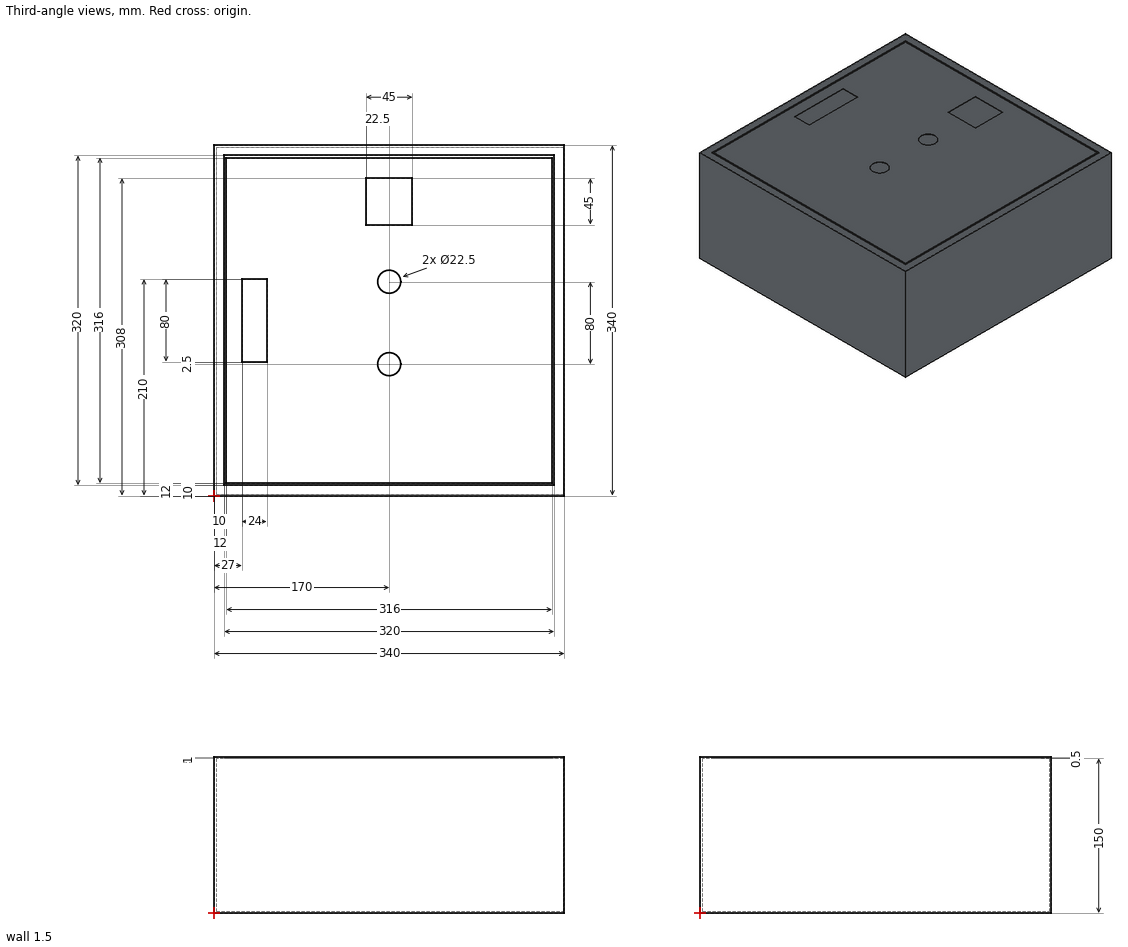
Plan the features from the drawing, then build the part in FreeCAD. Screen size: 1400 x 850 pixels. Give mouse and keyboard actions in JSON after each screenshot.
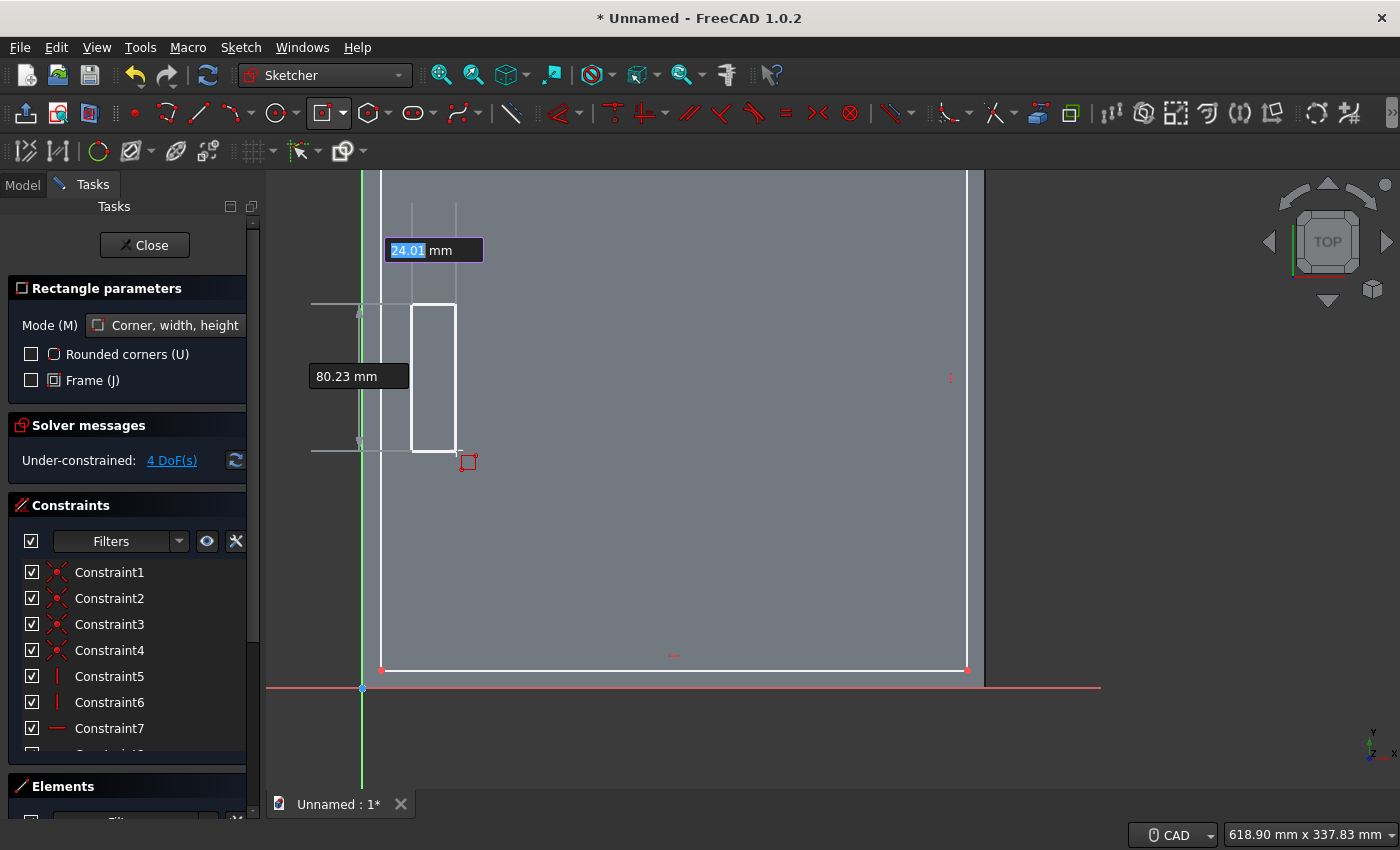
{"action": "type", "text": "24"}
{"action": "key", "text": "Tab"}
{"action": "type", "text": "80"}
{"action": "key", "text": "Return"}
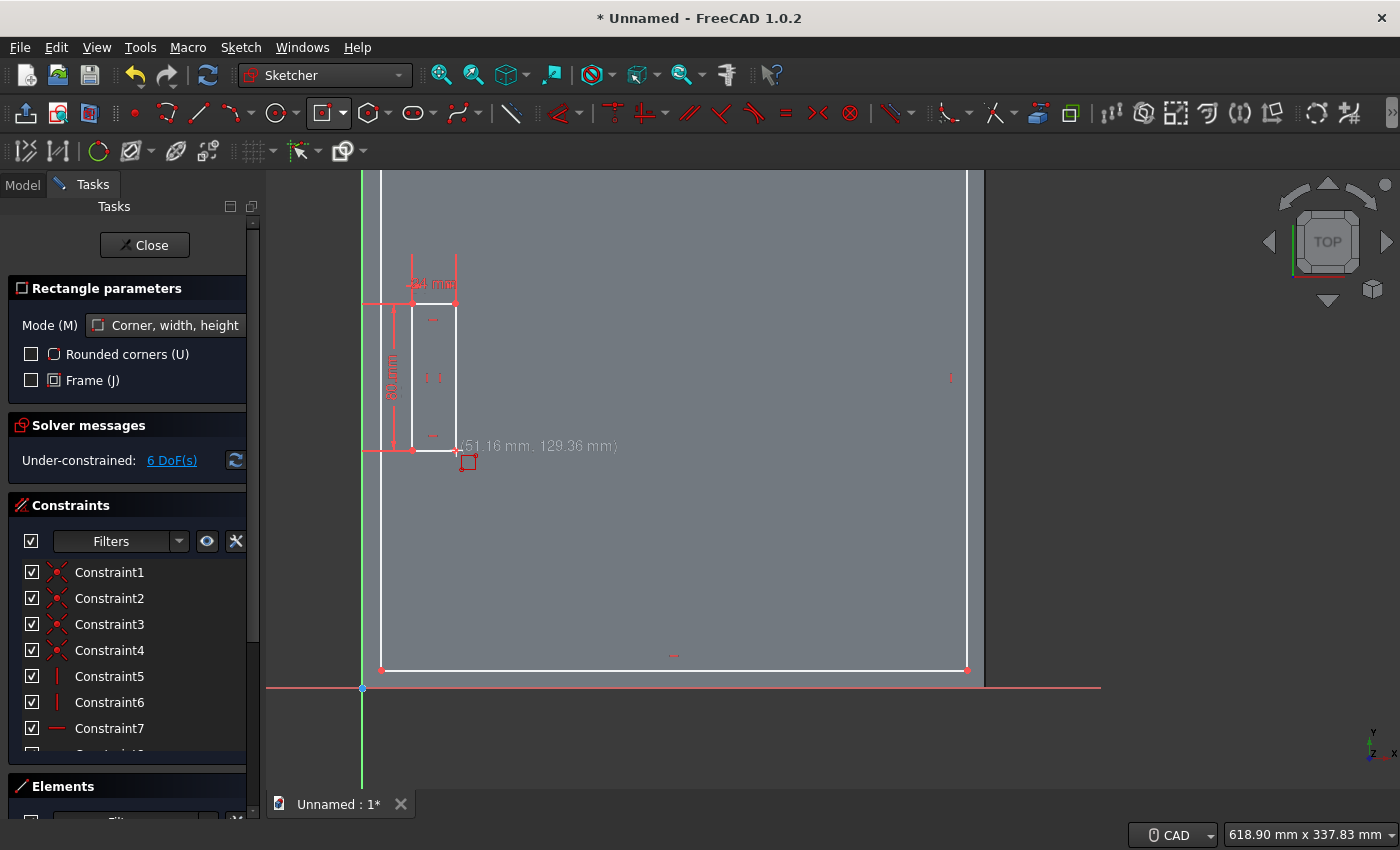
{"action": "scroll", "coordinate": [968, 670], "scroll_direction": "down", "scroll_amount": 2}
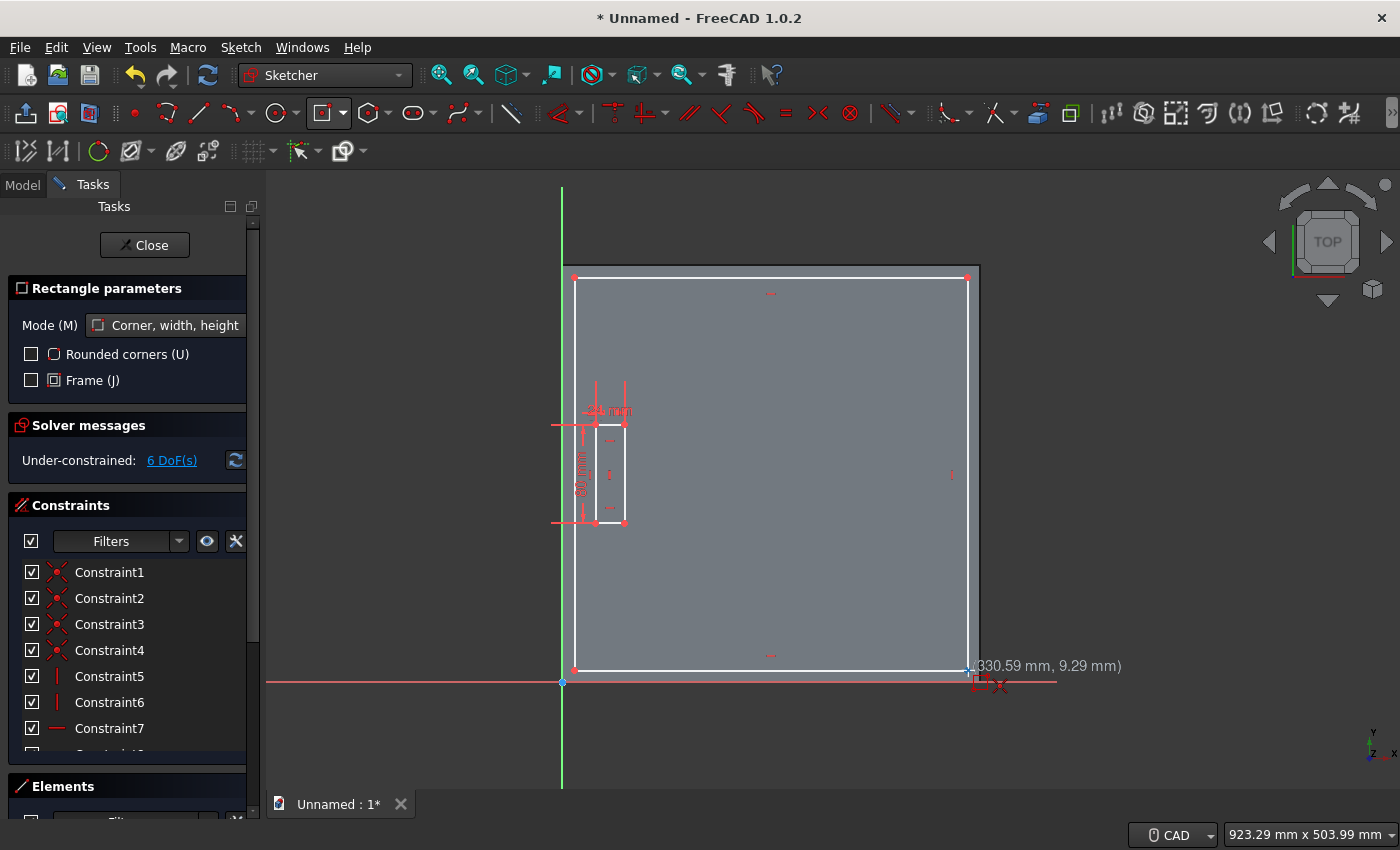
{"action": "left_click", "coordinate": [743, 304]}
{"action": "mouse_move", "coordinate": [799, 359]}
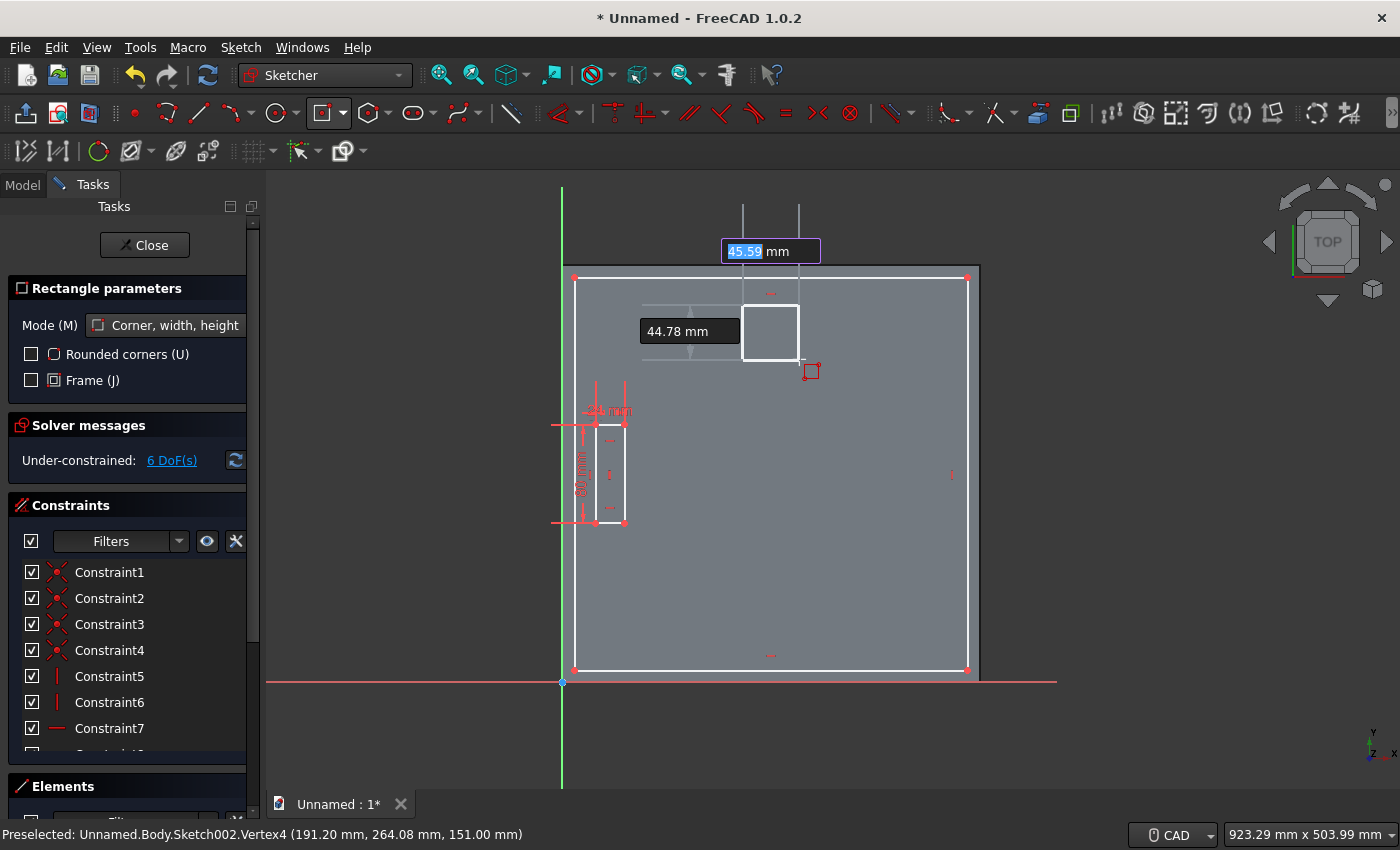
{"action": "type", "text": "45"}
{"action": "key", "text": "Tab"}
{"action": "type", "text": "45"}
{"action": "key", "text": "Return"}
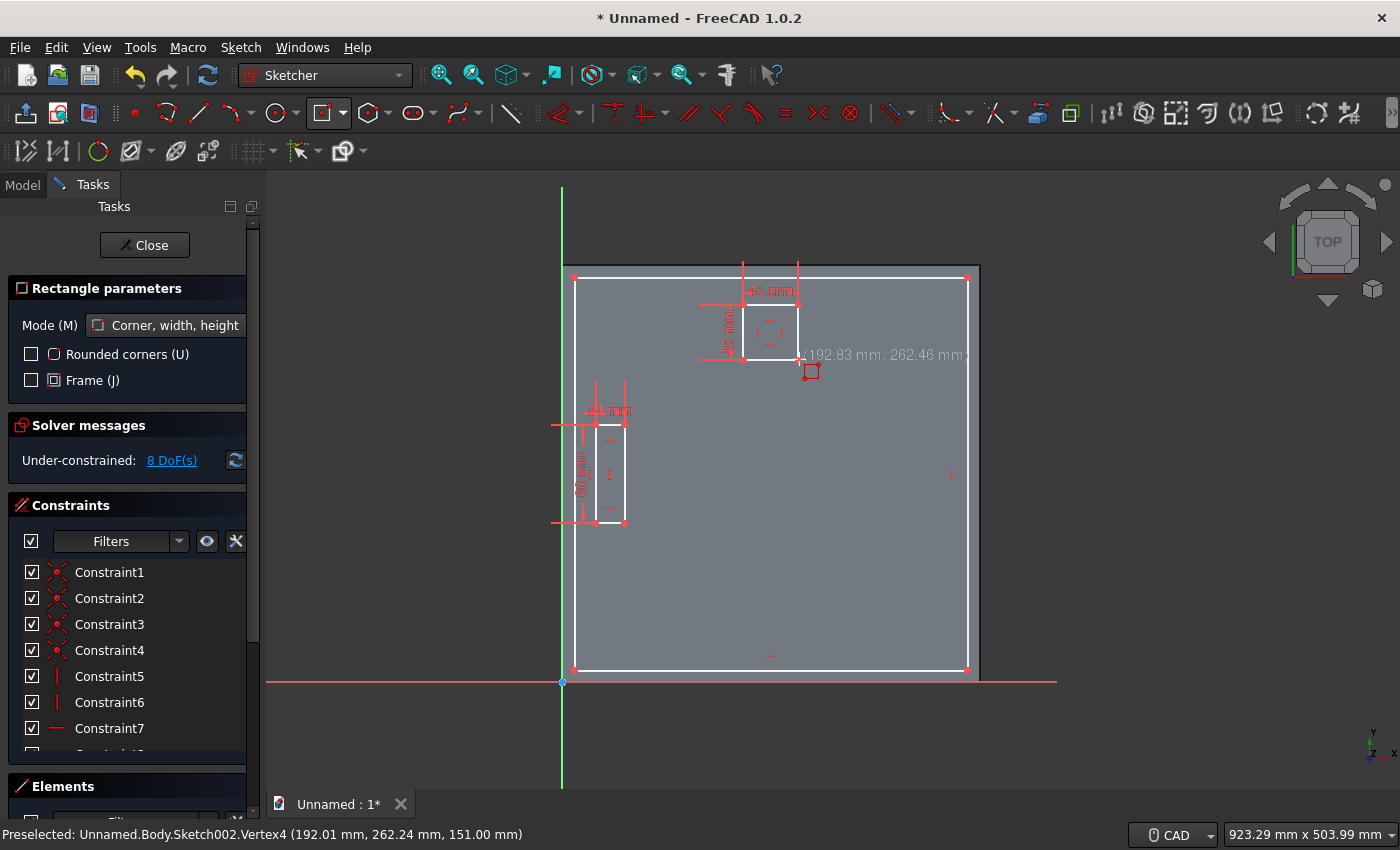
{"action": "scroll", "coordinate": [577, 279], "scroll_direction": "up", "scroll_amount": 10}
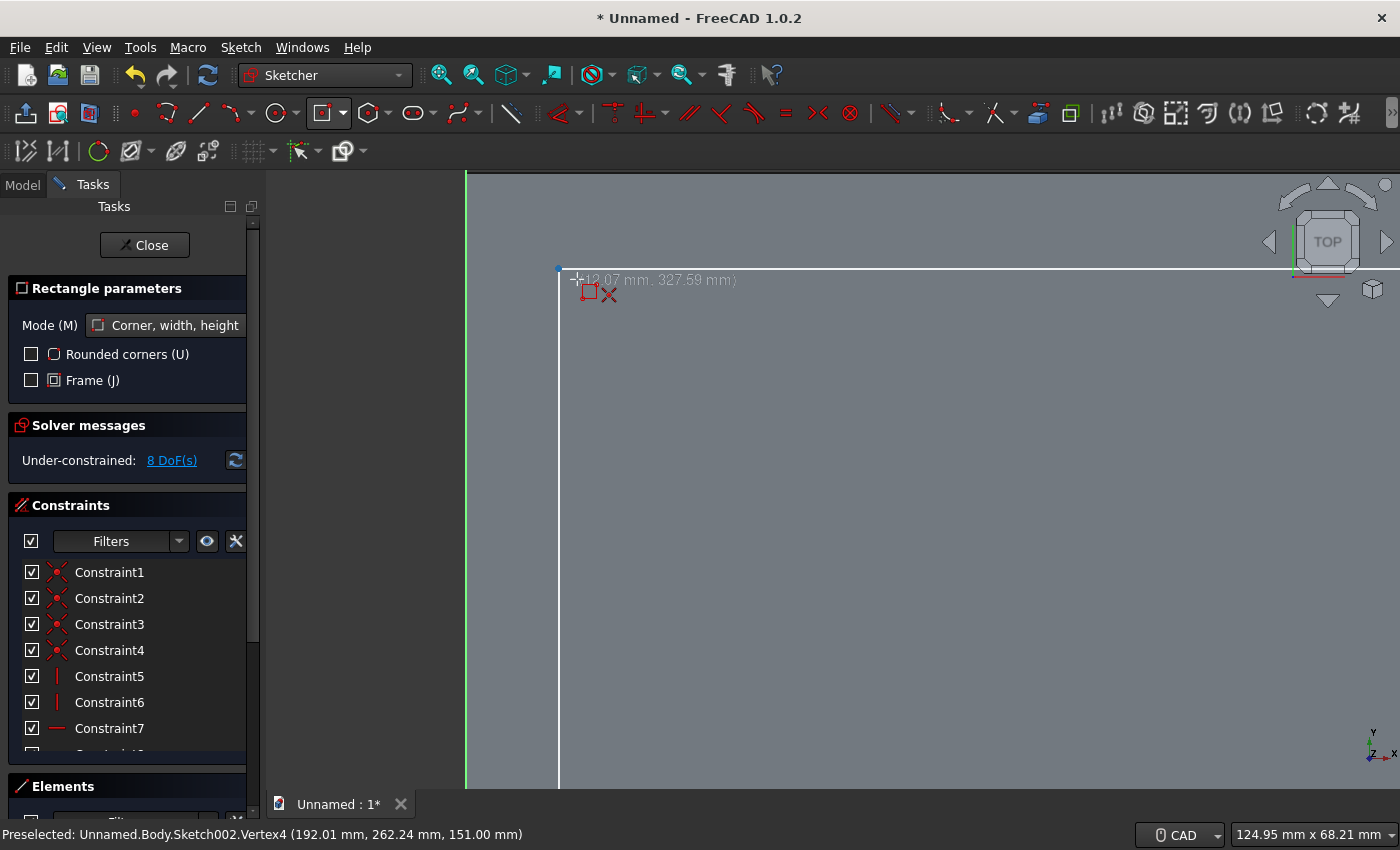
{"action": "left_click", "coordinate": [575, 282]}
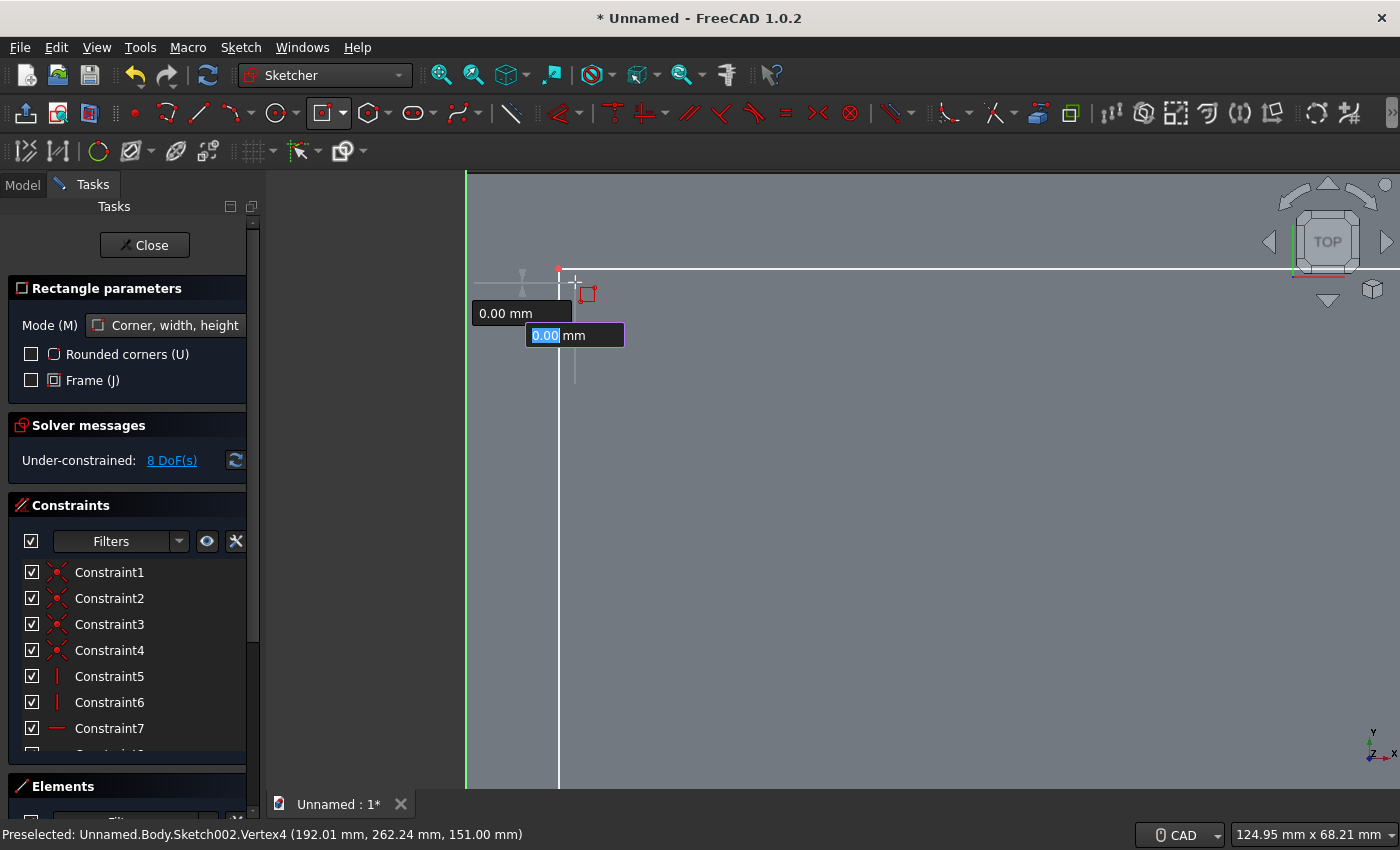
{"action": "scroll", "coordinate": [577, 279], "scroll_direction": "down", "scroll_amount": 10}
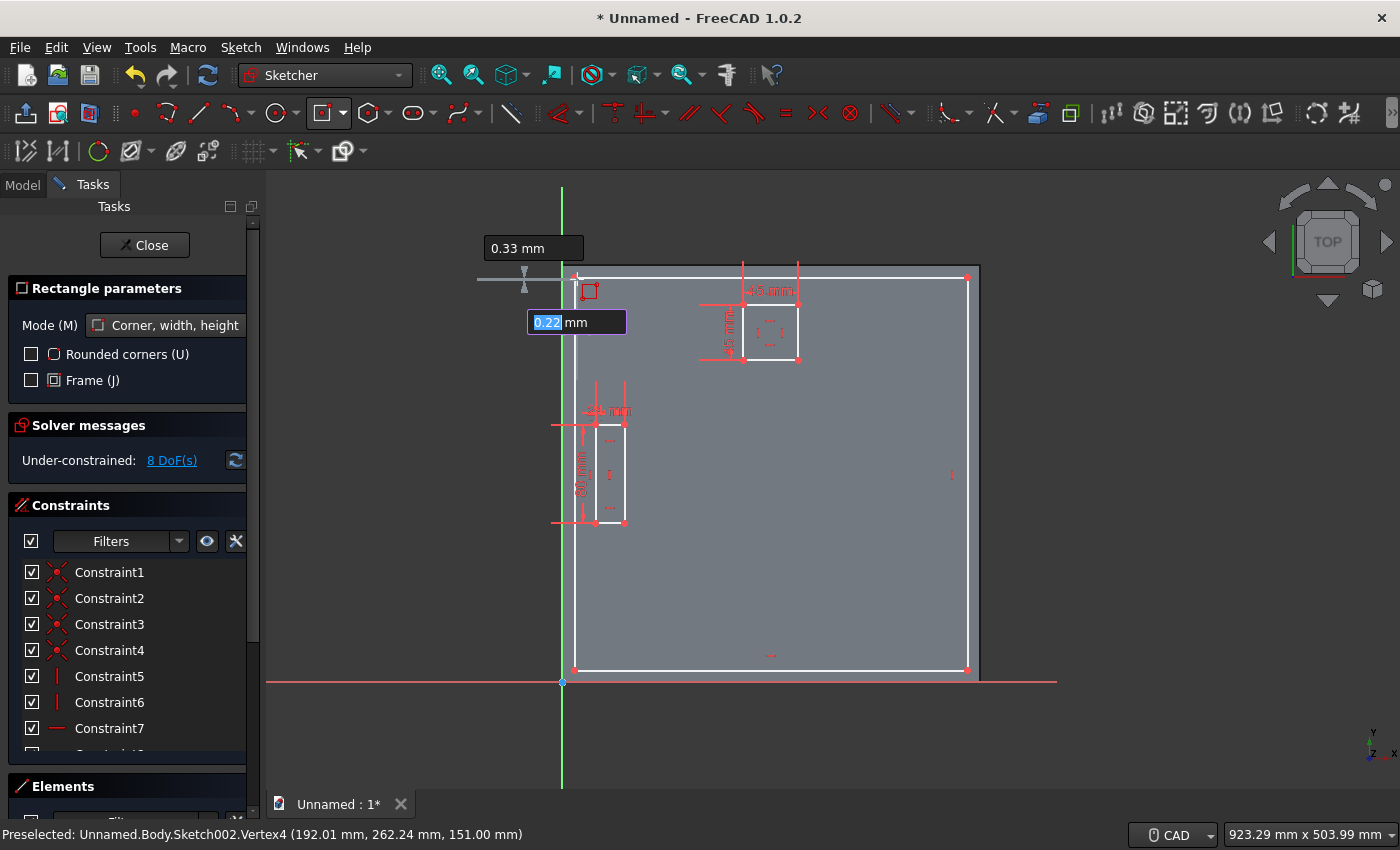
{"action": "scroll", "coordinate": [965, 668], "scroll_direction": "up", "scroll_amount": 10}